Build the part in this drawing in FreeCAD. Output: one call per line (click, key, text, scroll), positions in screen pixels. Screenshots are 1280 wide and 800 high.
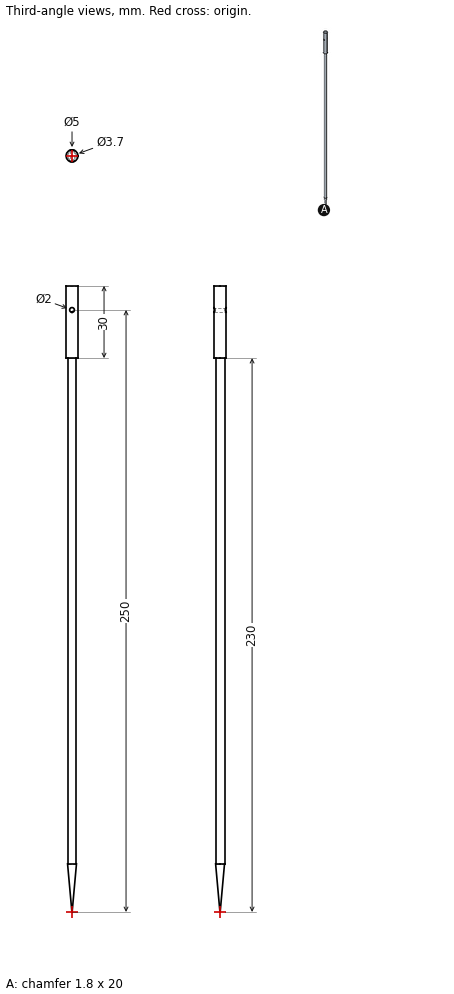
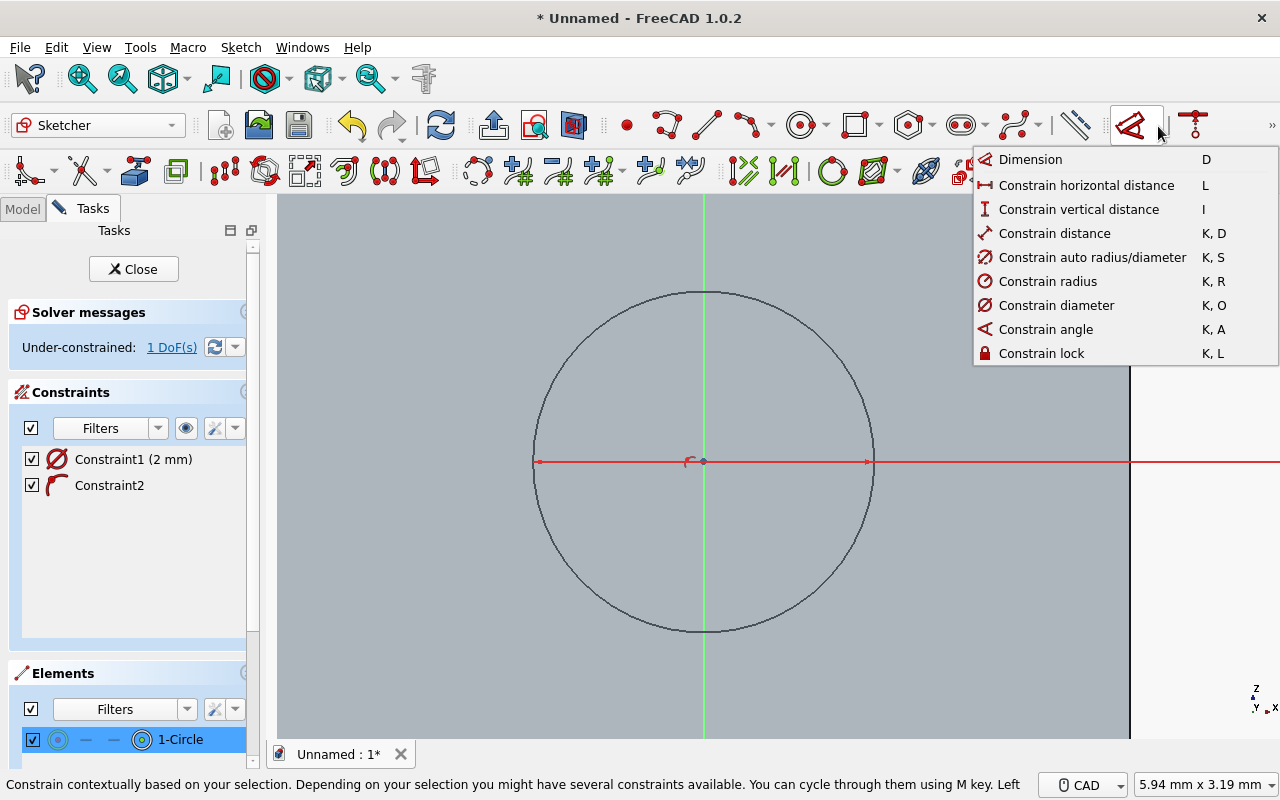
click(1126, 209)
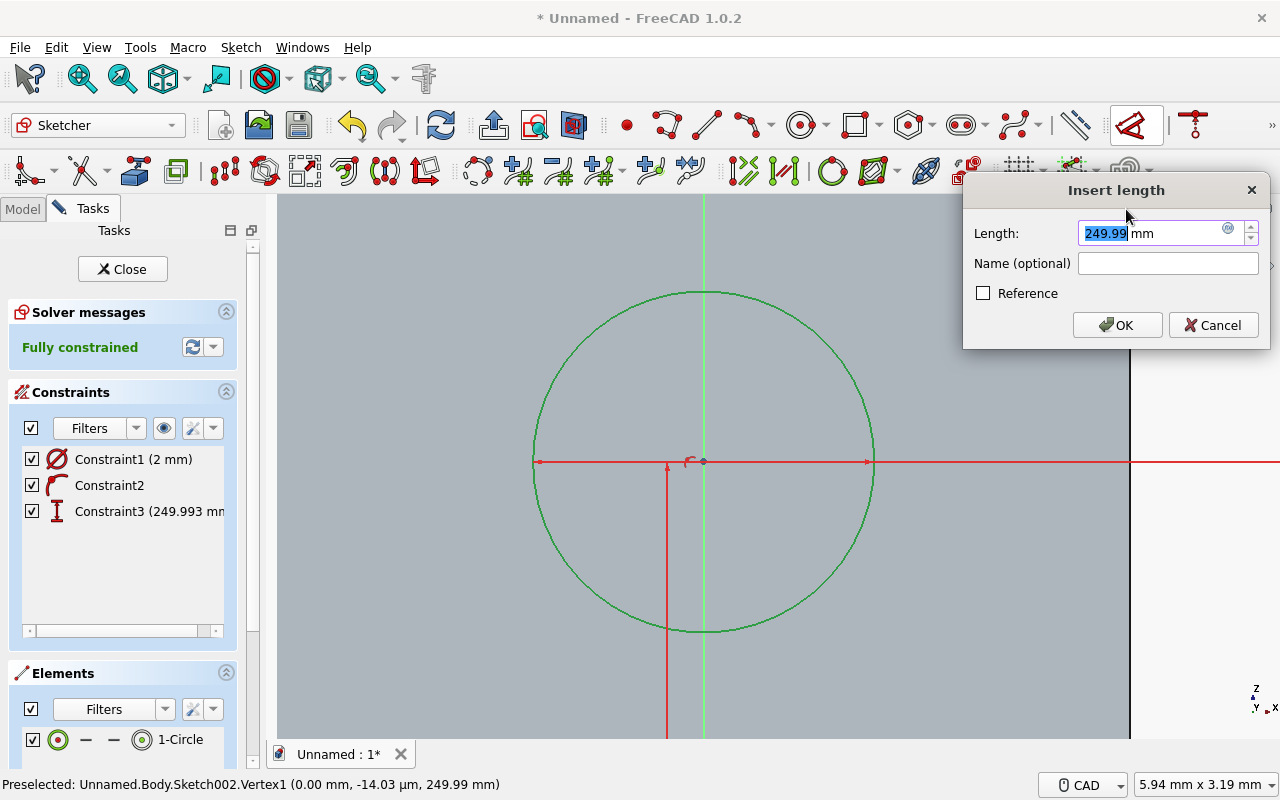
text(250)
key(Return)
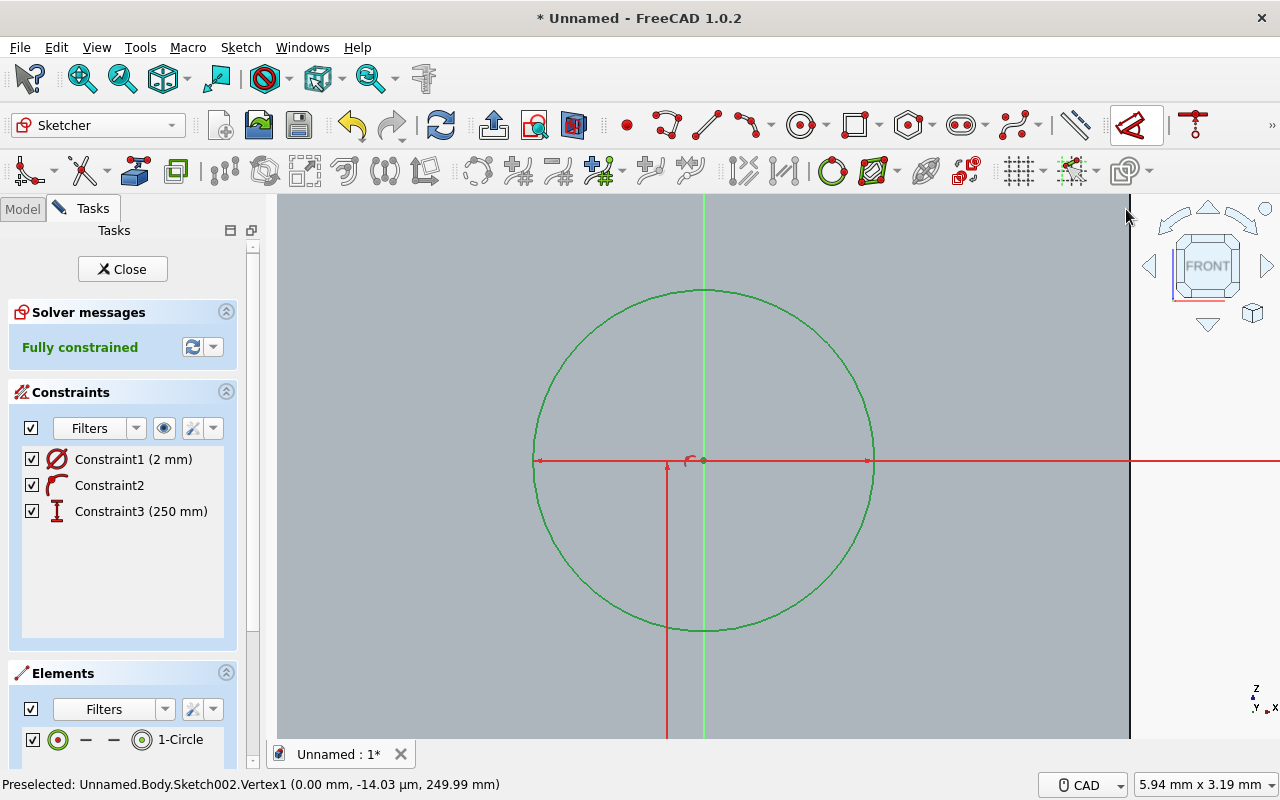
click(123, 269)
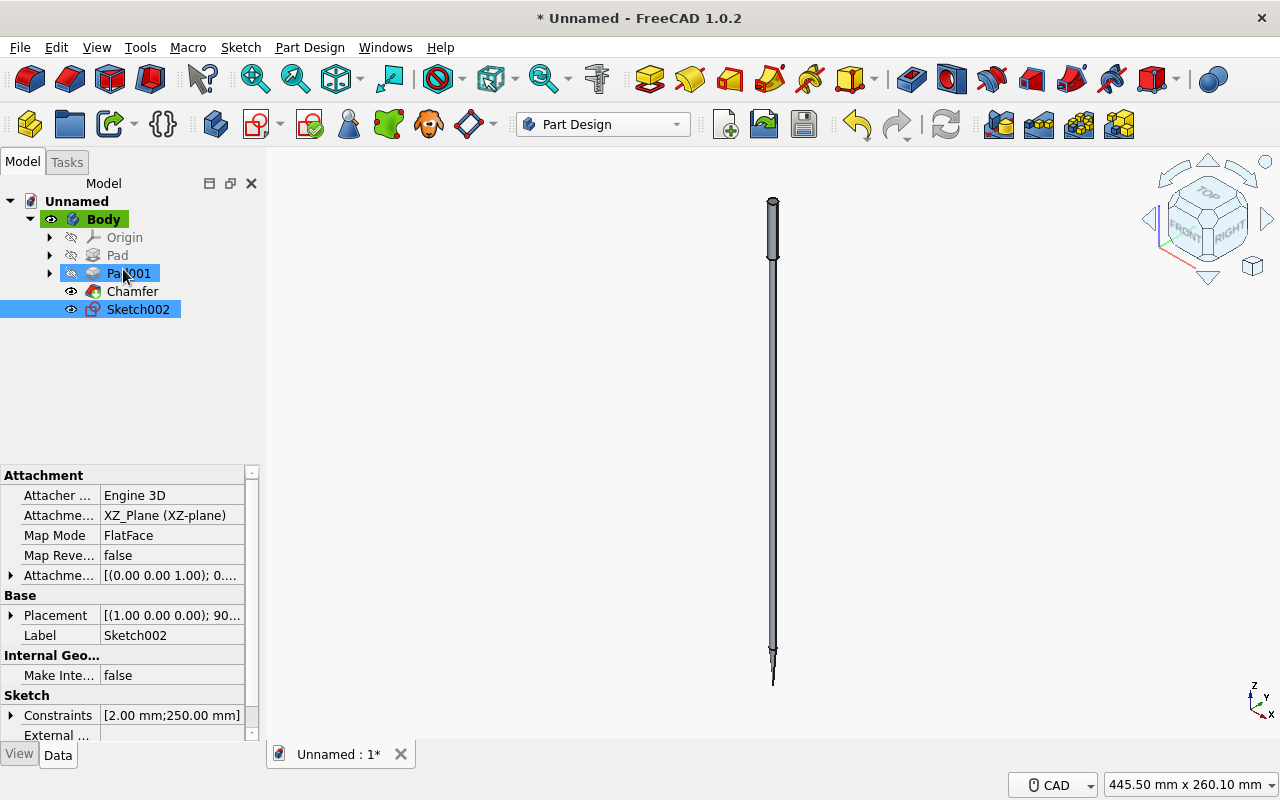
click(912, 80)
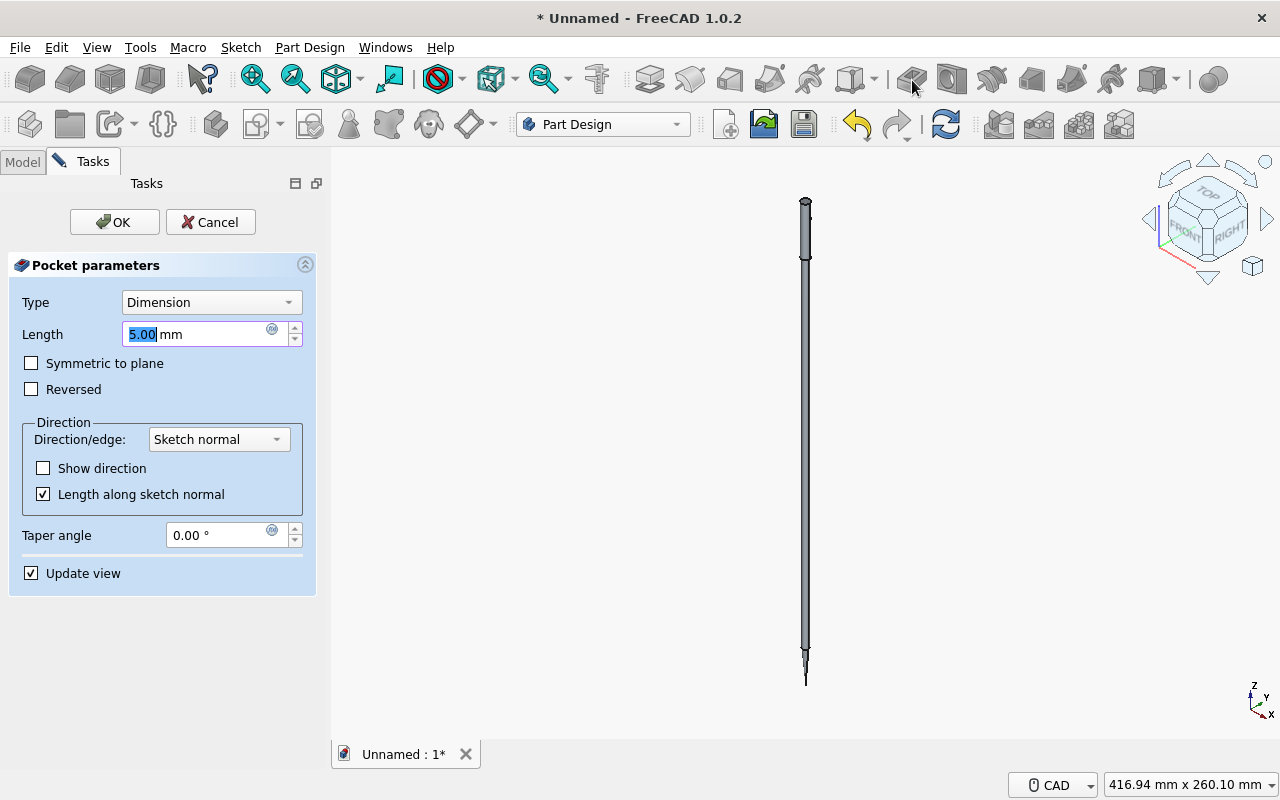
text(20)
key(Tab)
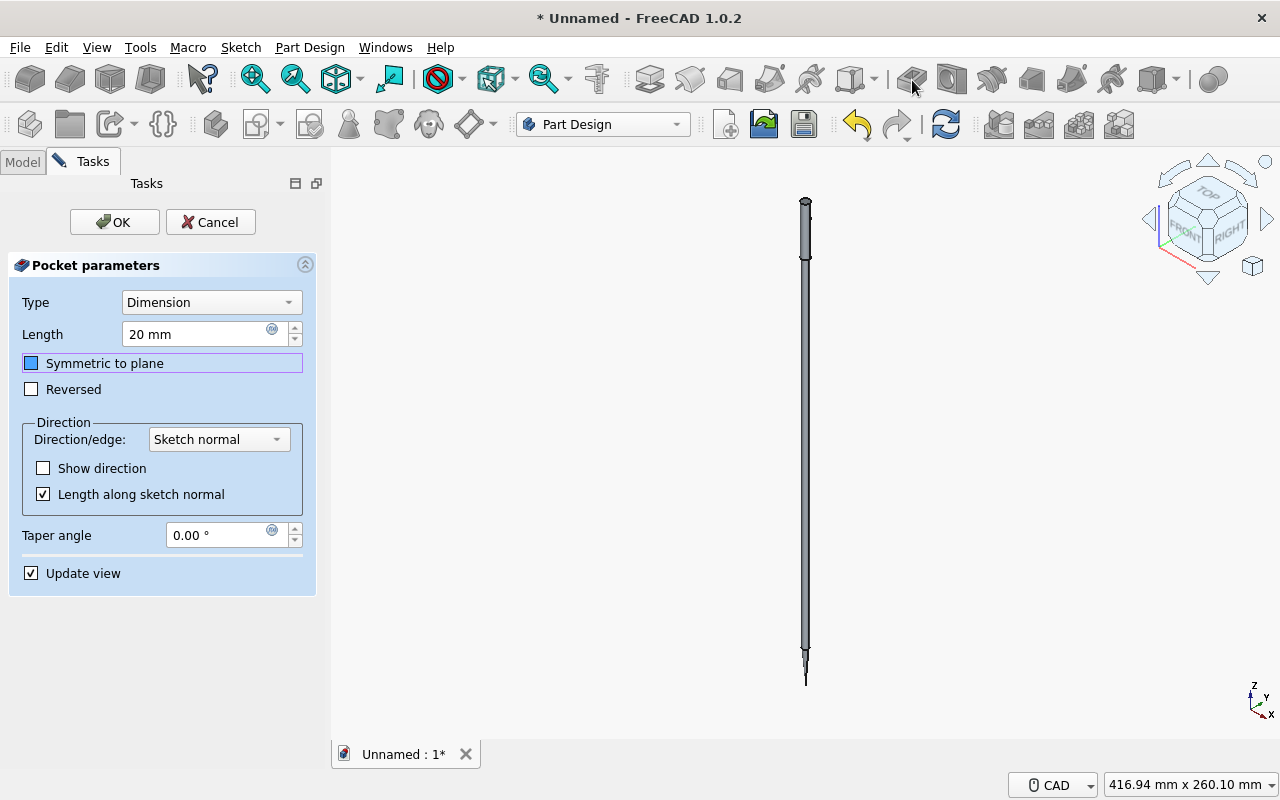
click(30, 363)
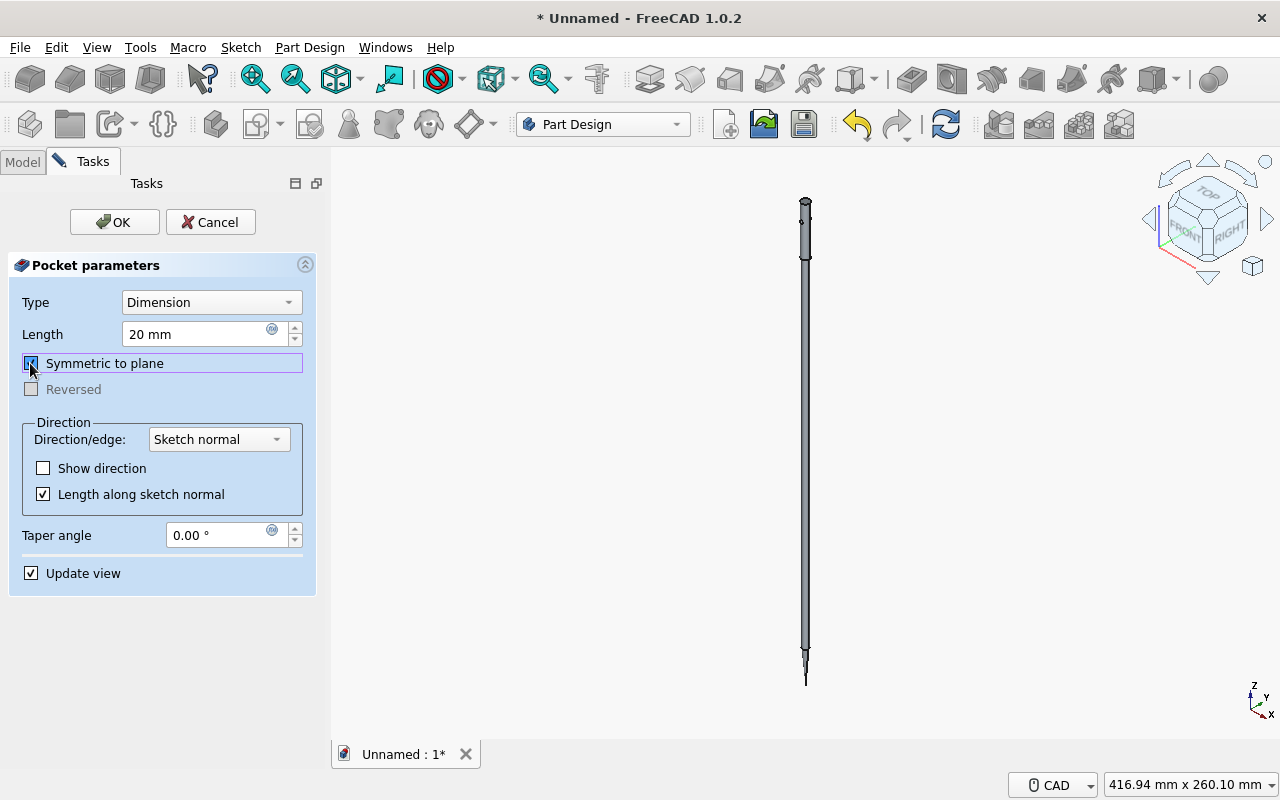
click(115, 222)